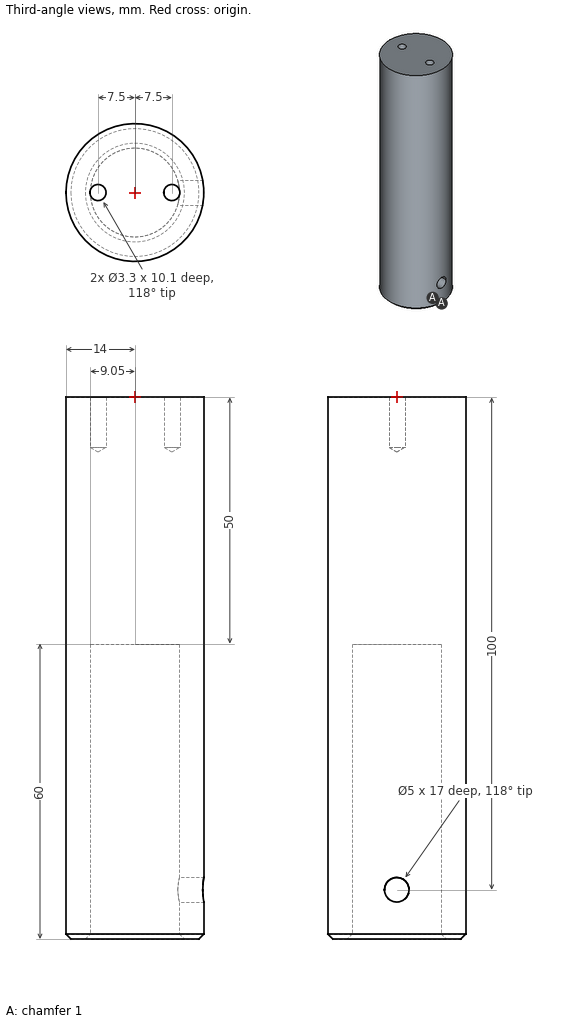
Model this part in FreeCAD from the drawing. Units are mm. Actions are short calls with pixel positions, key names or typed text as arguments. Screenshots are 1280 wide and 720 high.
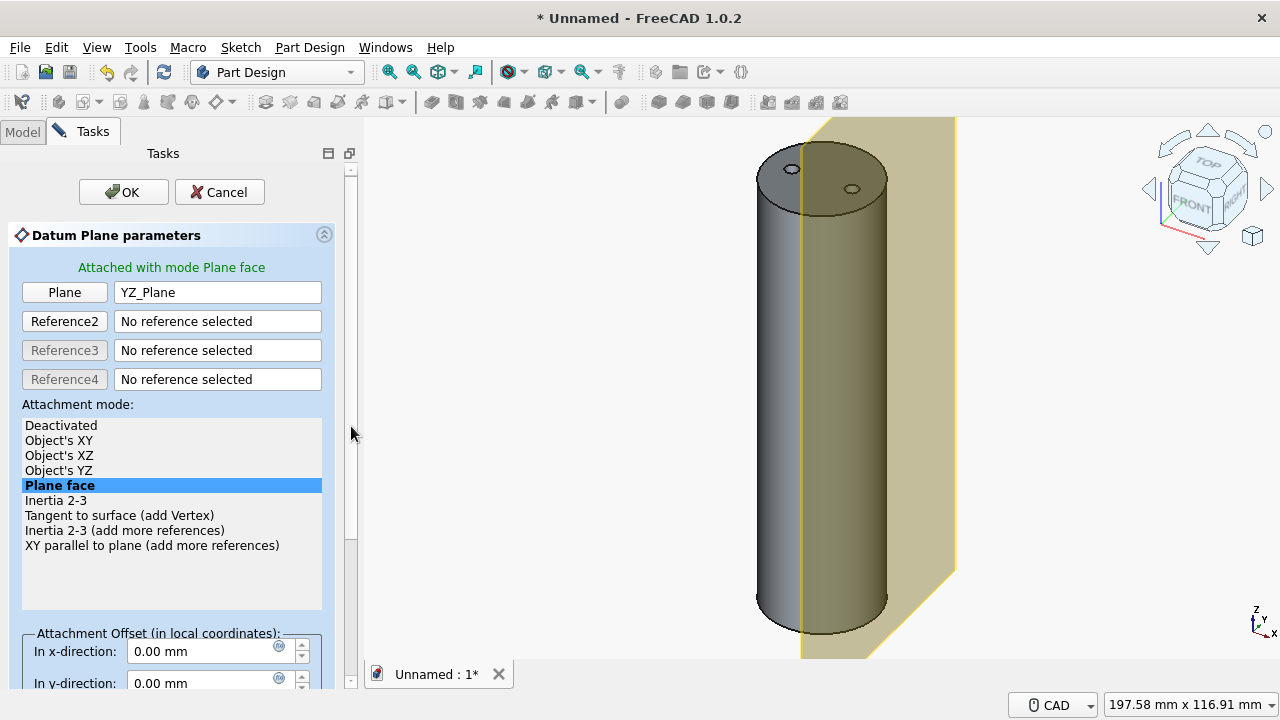
click(124, 192)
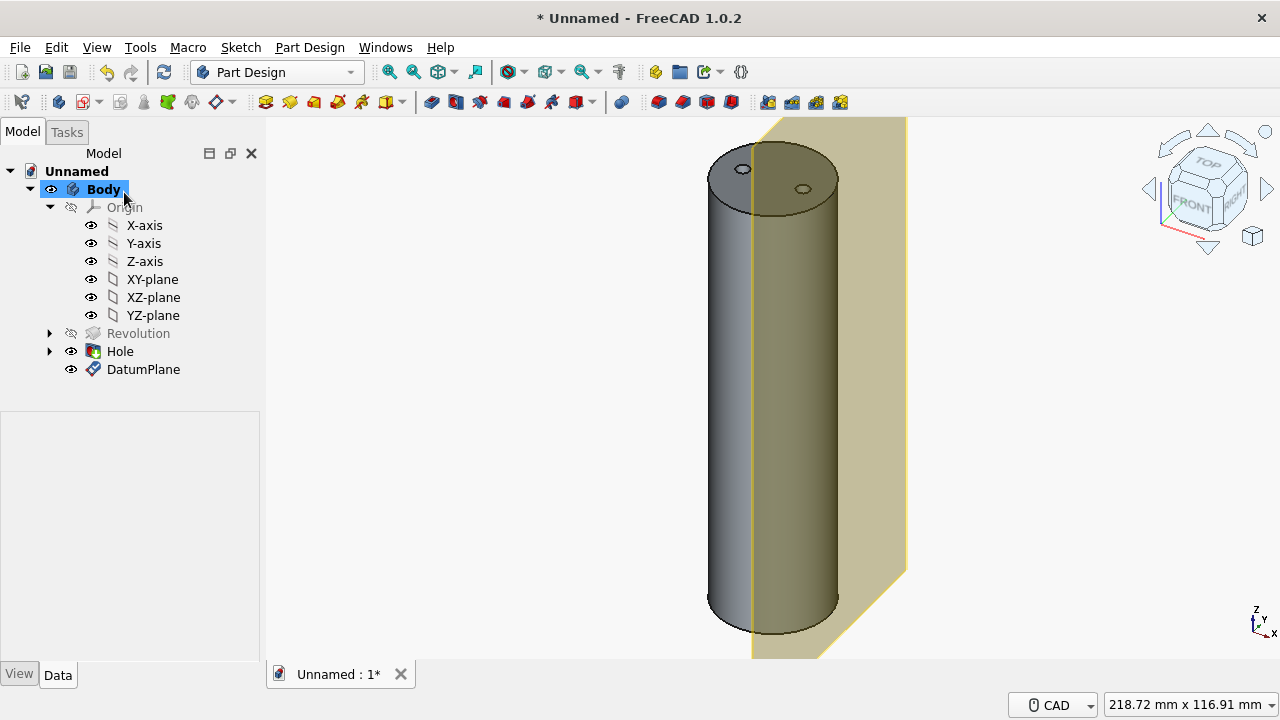
click(116, 369)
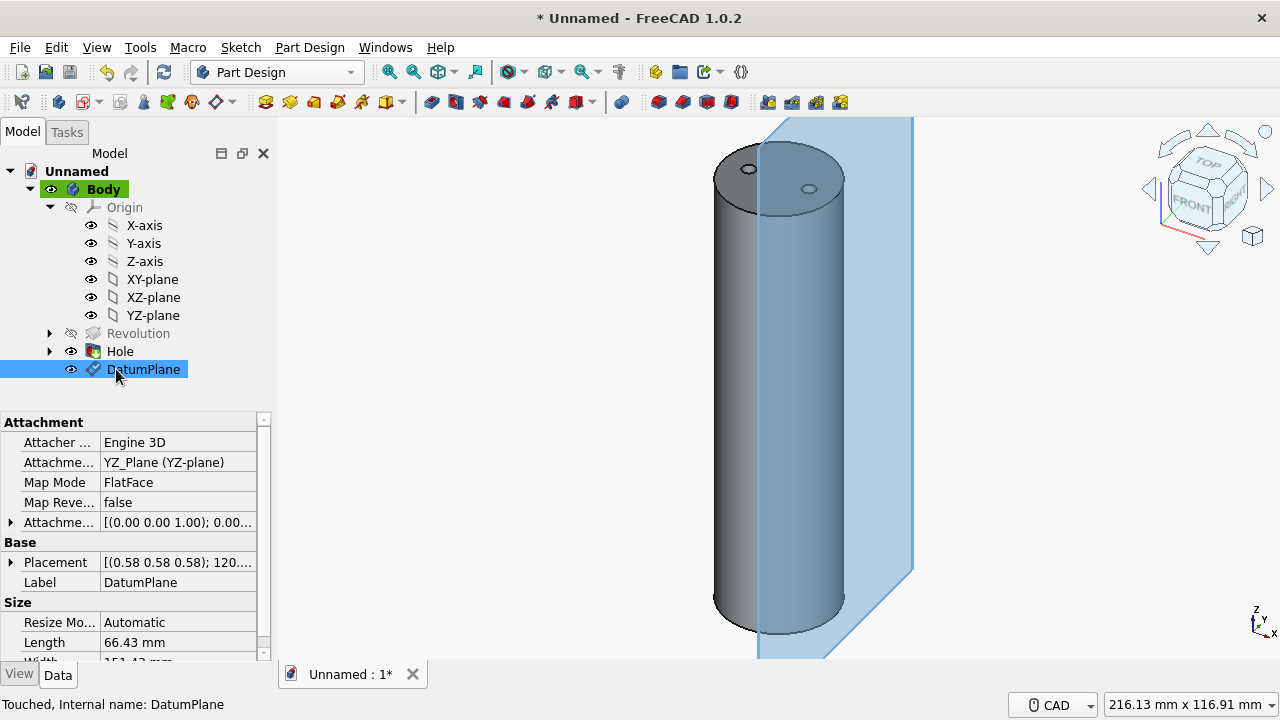
click(84, 102)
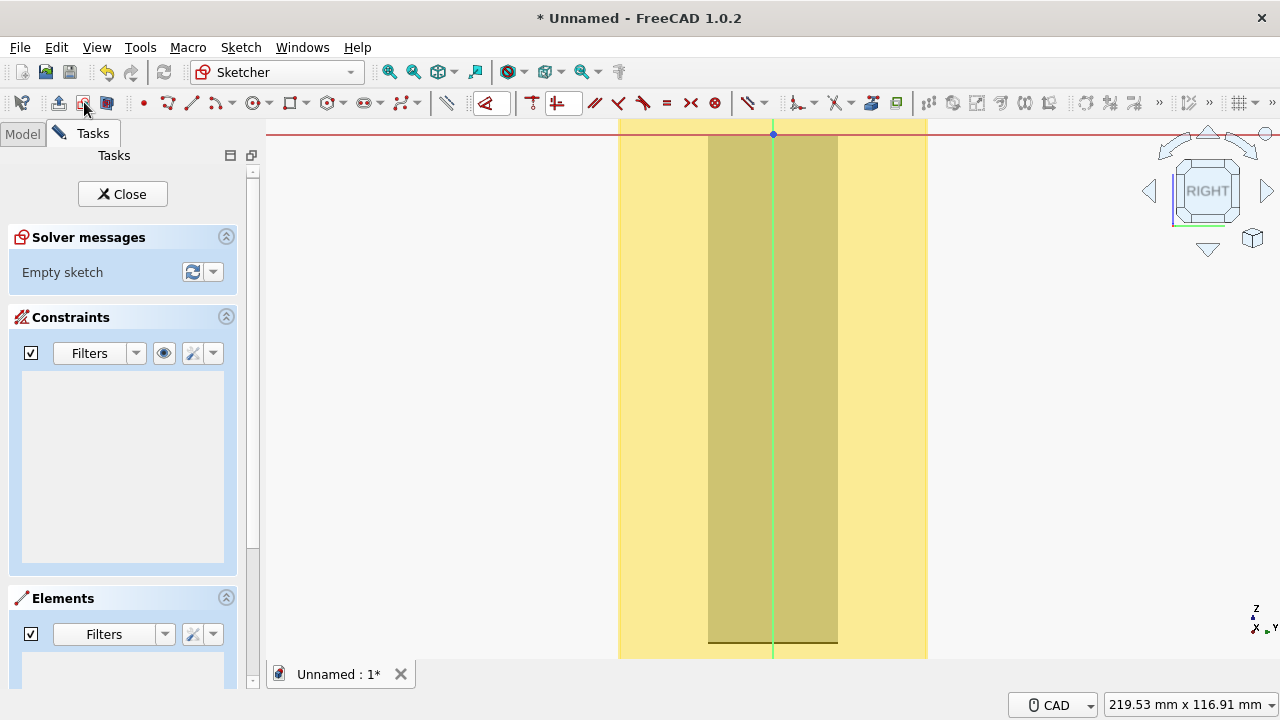
scroll(778, 614, up, 13)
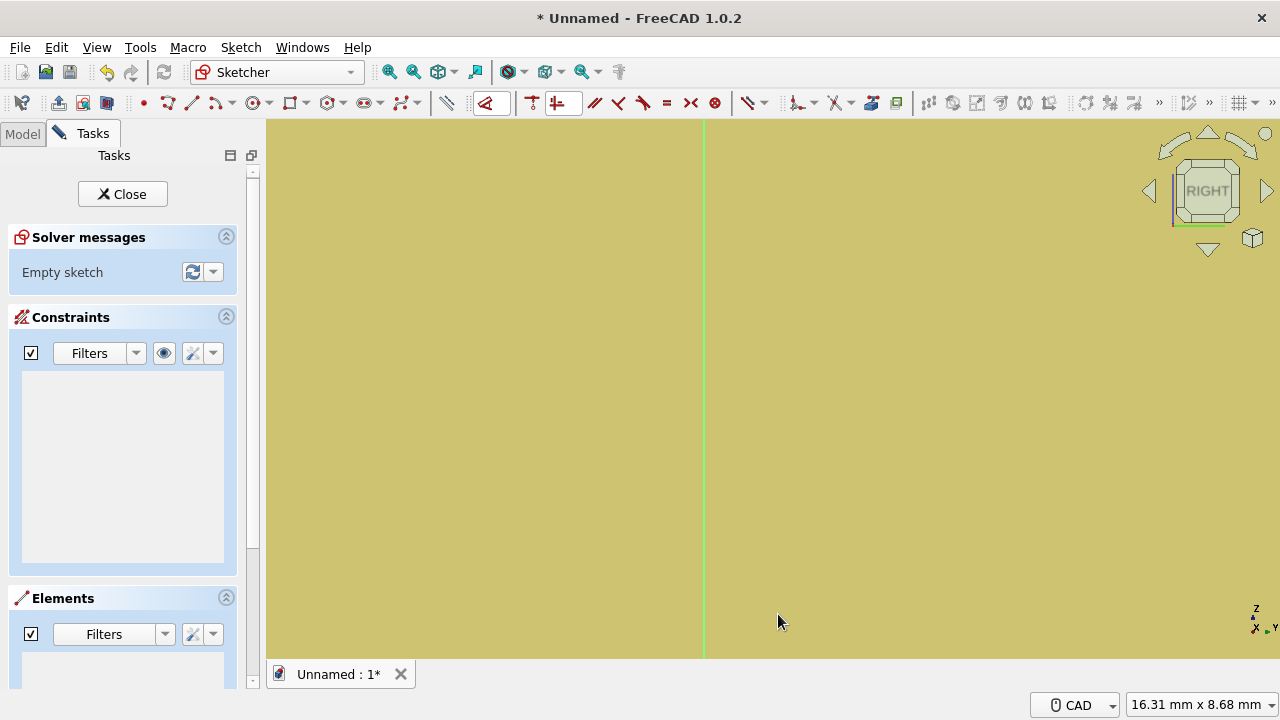
click(254, 104)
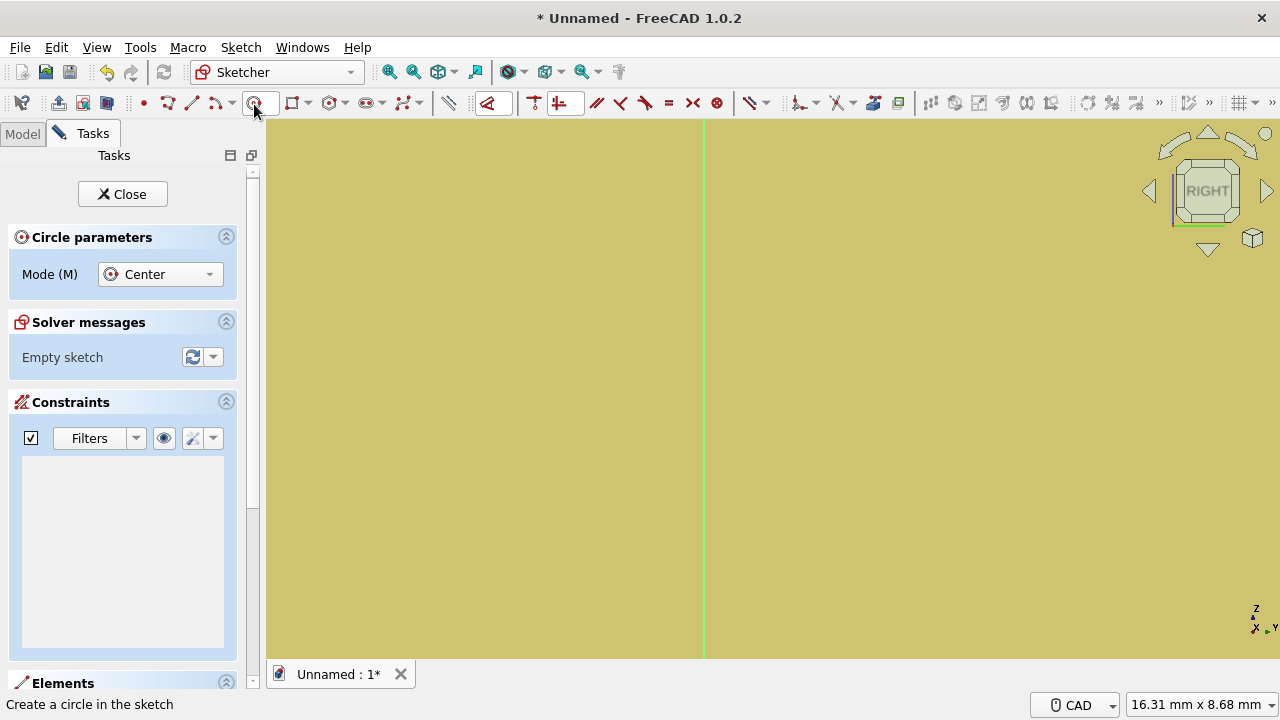
click(704, 372)
click(814, 262)
key(Escape)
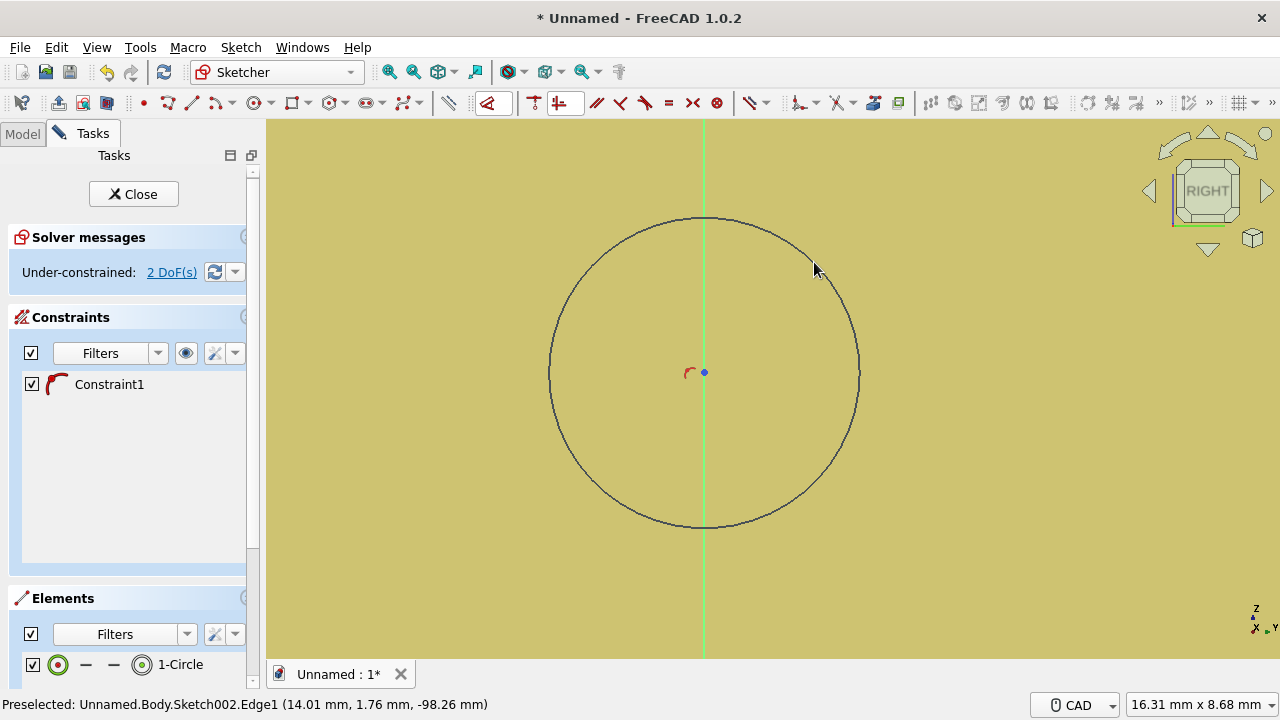
click(814, 263)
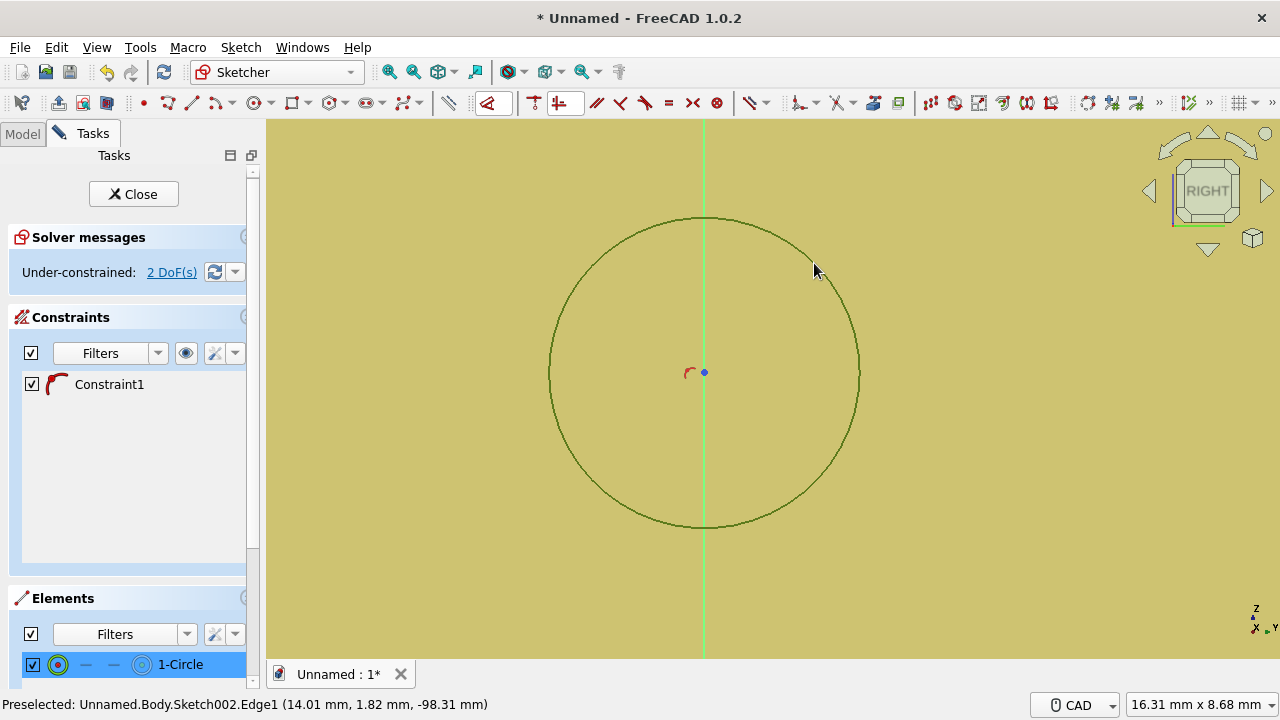
click(506, 104)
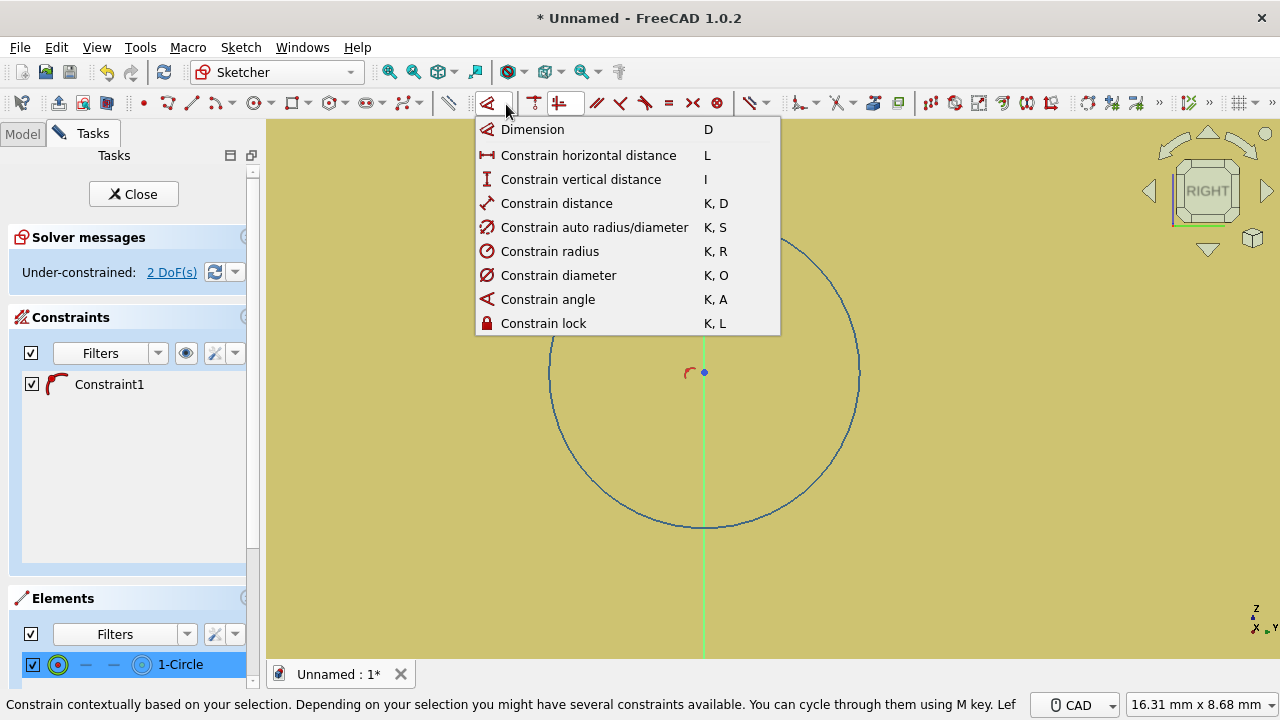
click(628, 275)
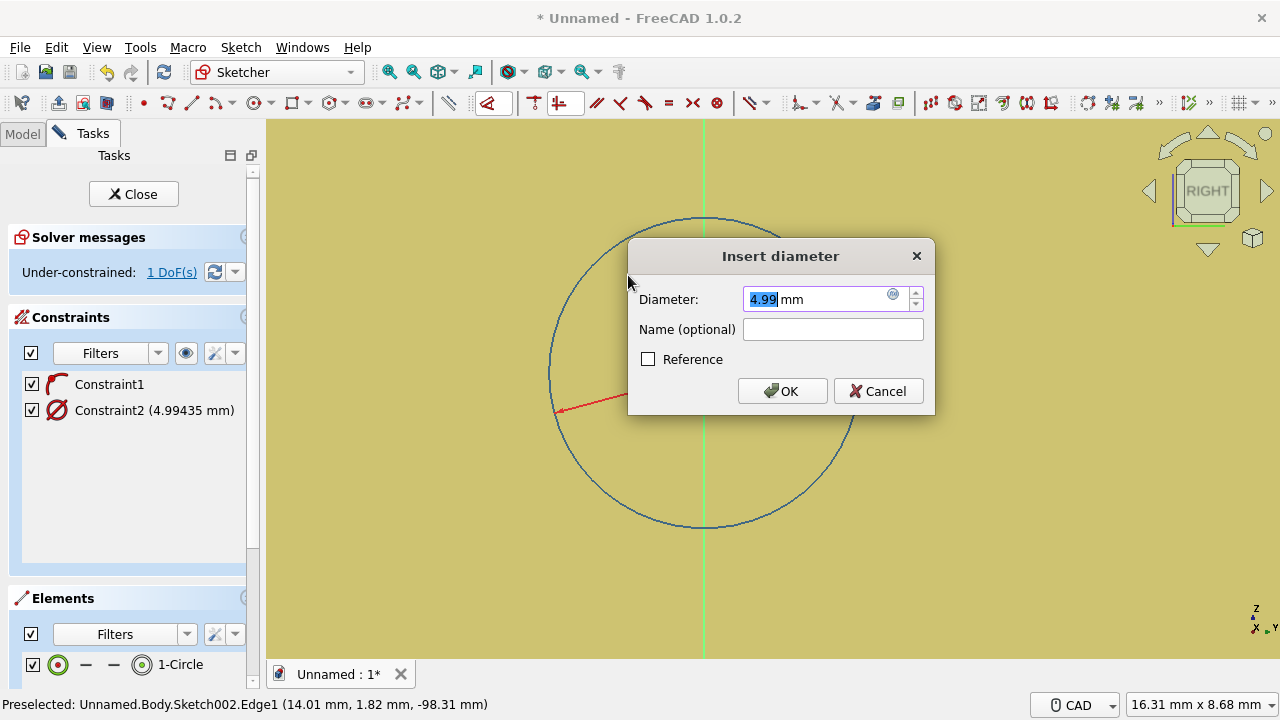
text(5)
key(Return)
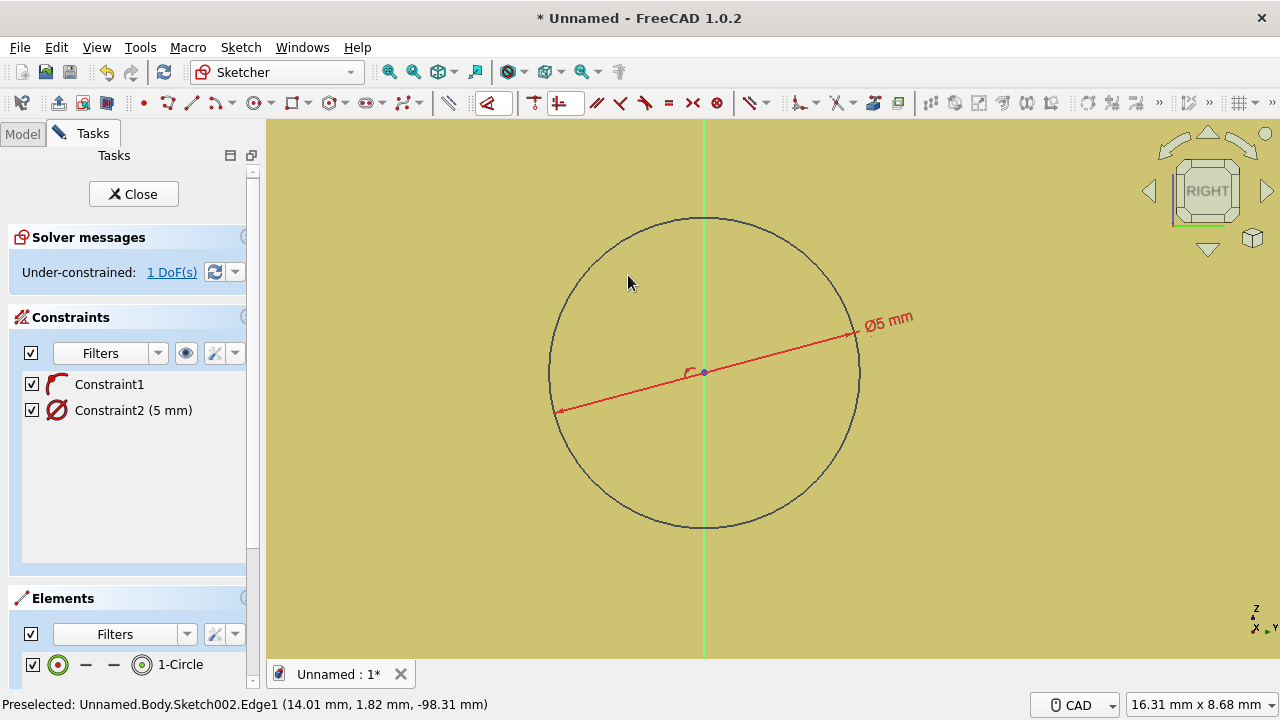
click(704, 373)